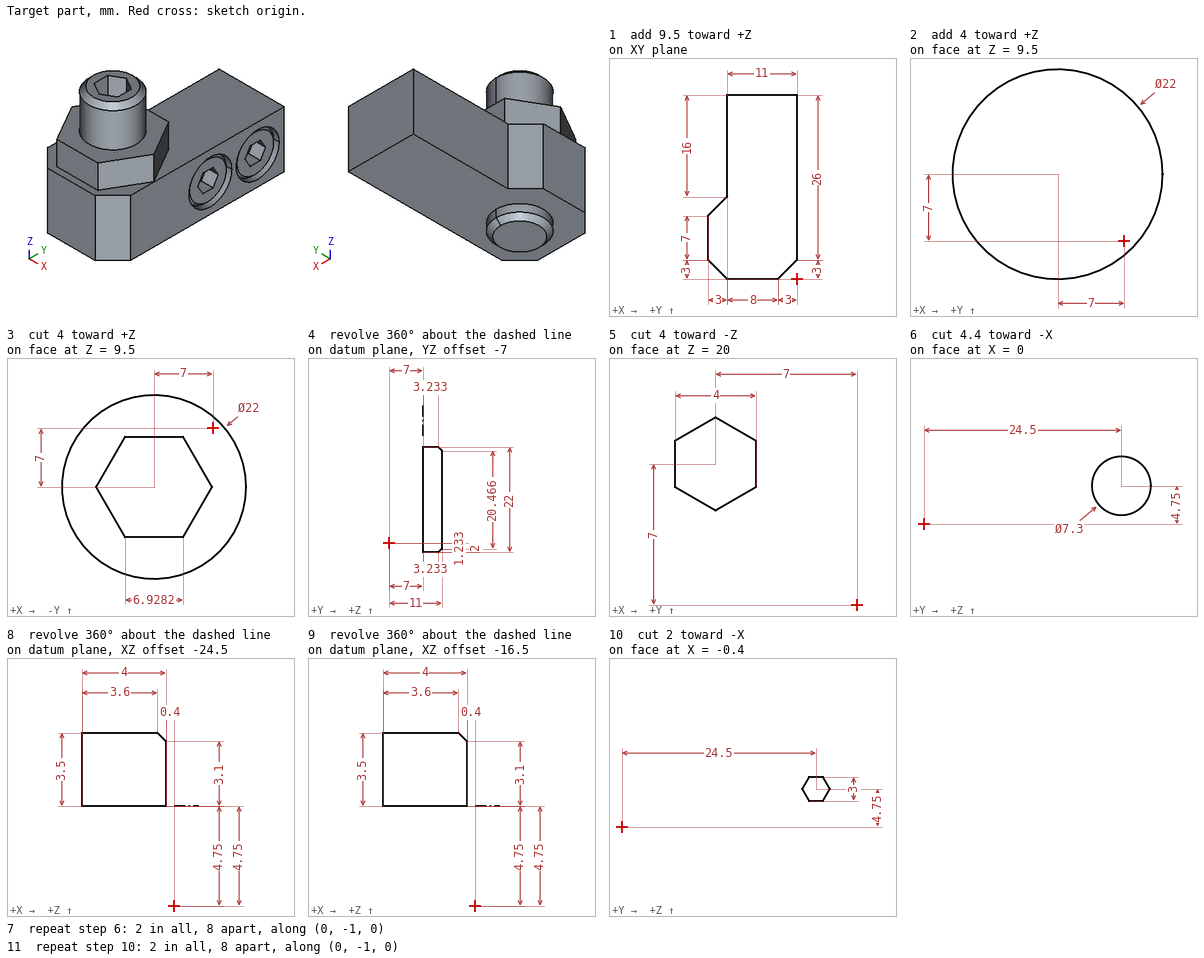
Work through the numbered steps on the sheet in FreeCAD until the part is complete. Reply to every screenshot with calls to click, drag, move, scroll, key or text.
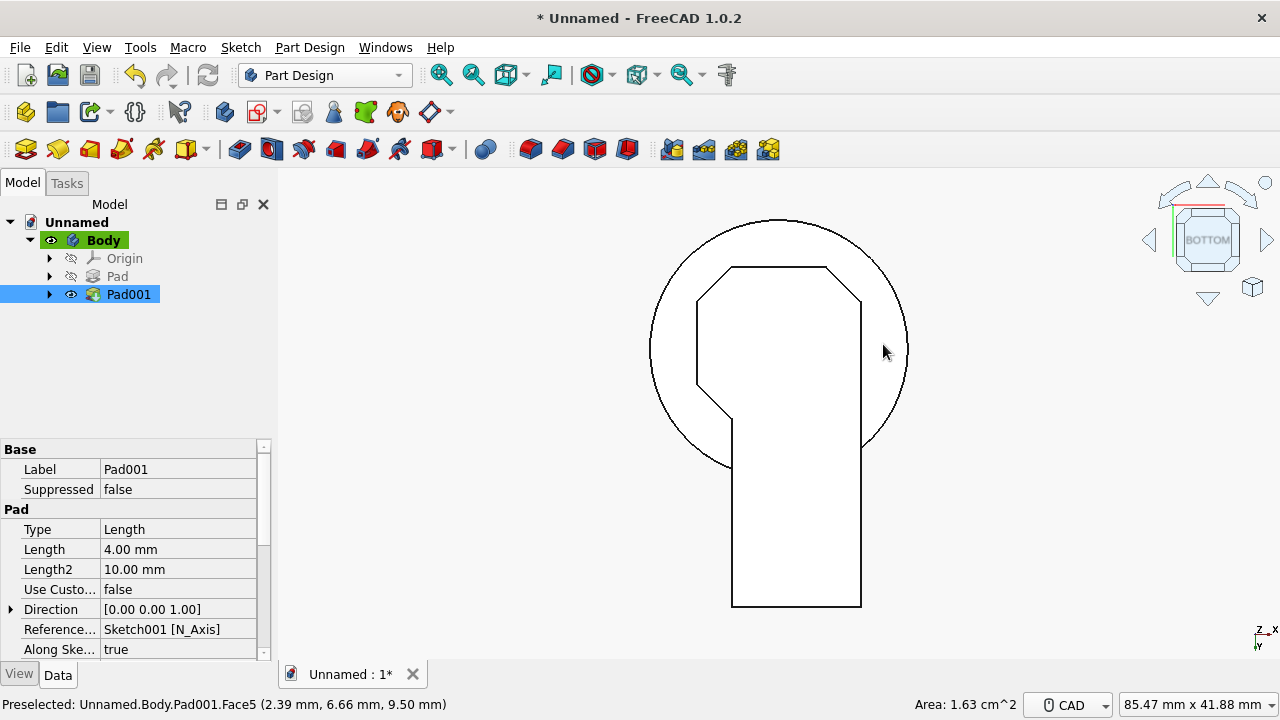
click(258, 112)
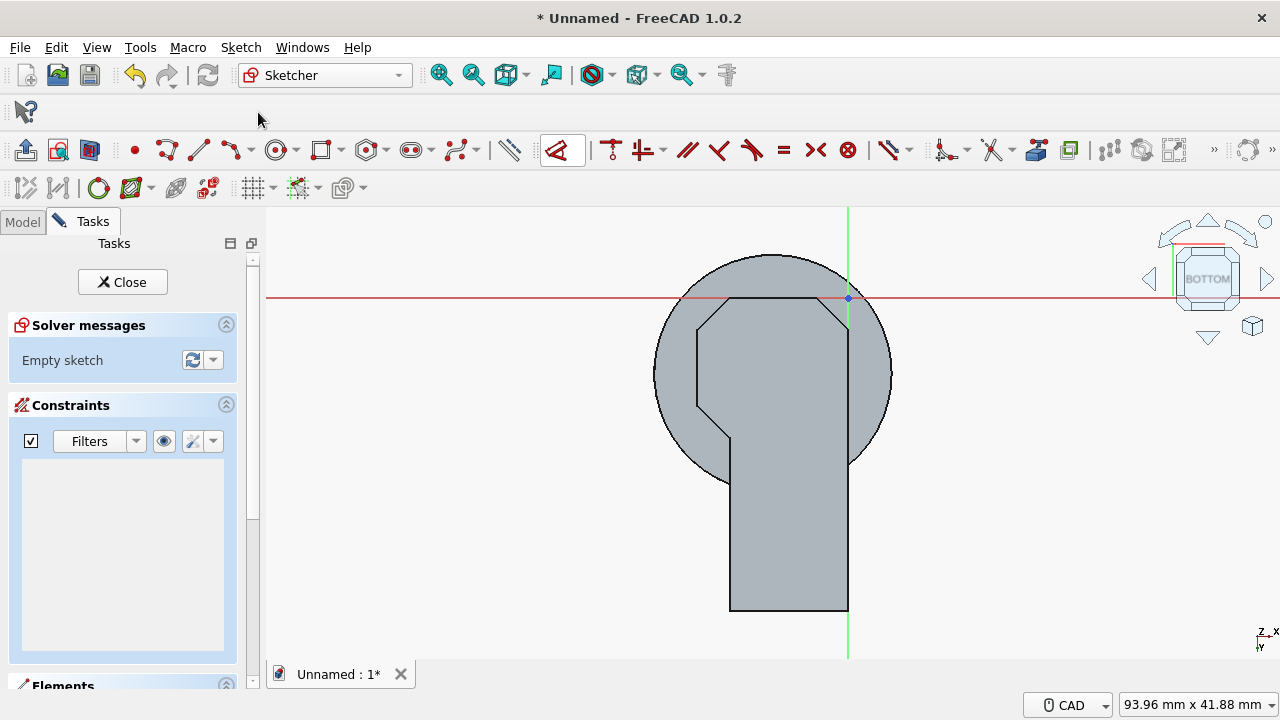
scroll(395, 631, down, 1)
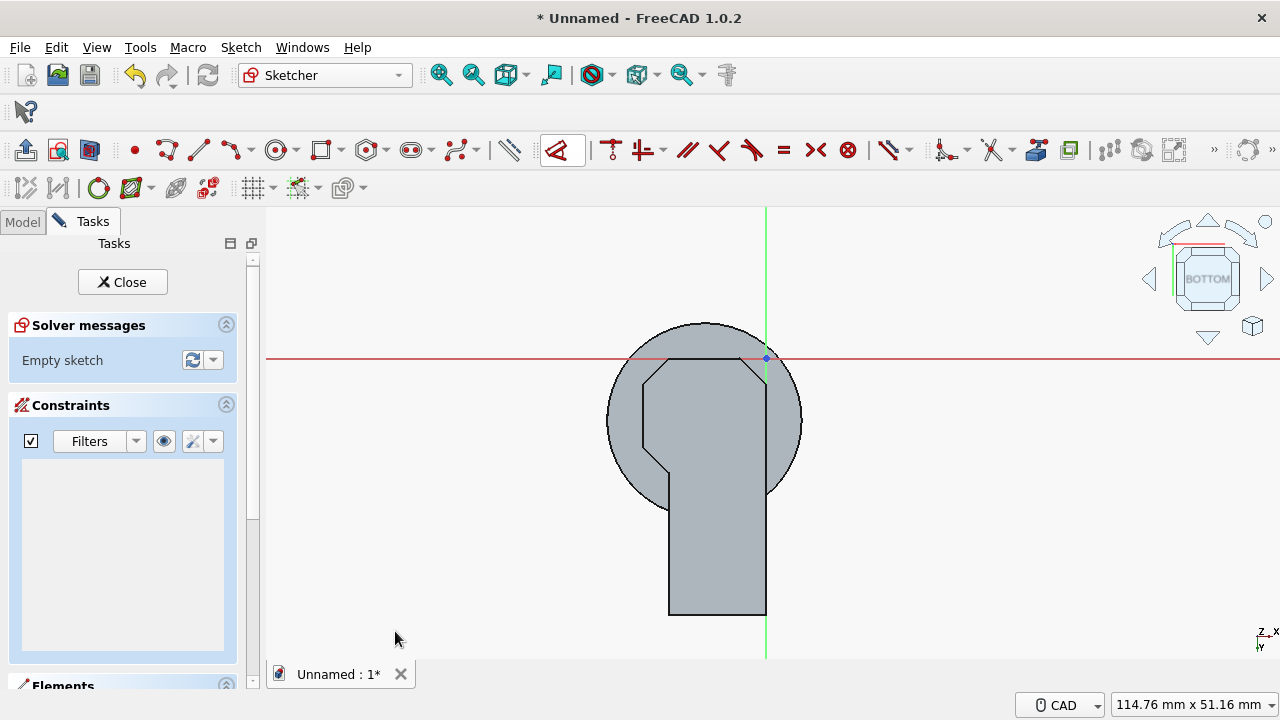
scroll(704, 395, up, 2)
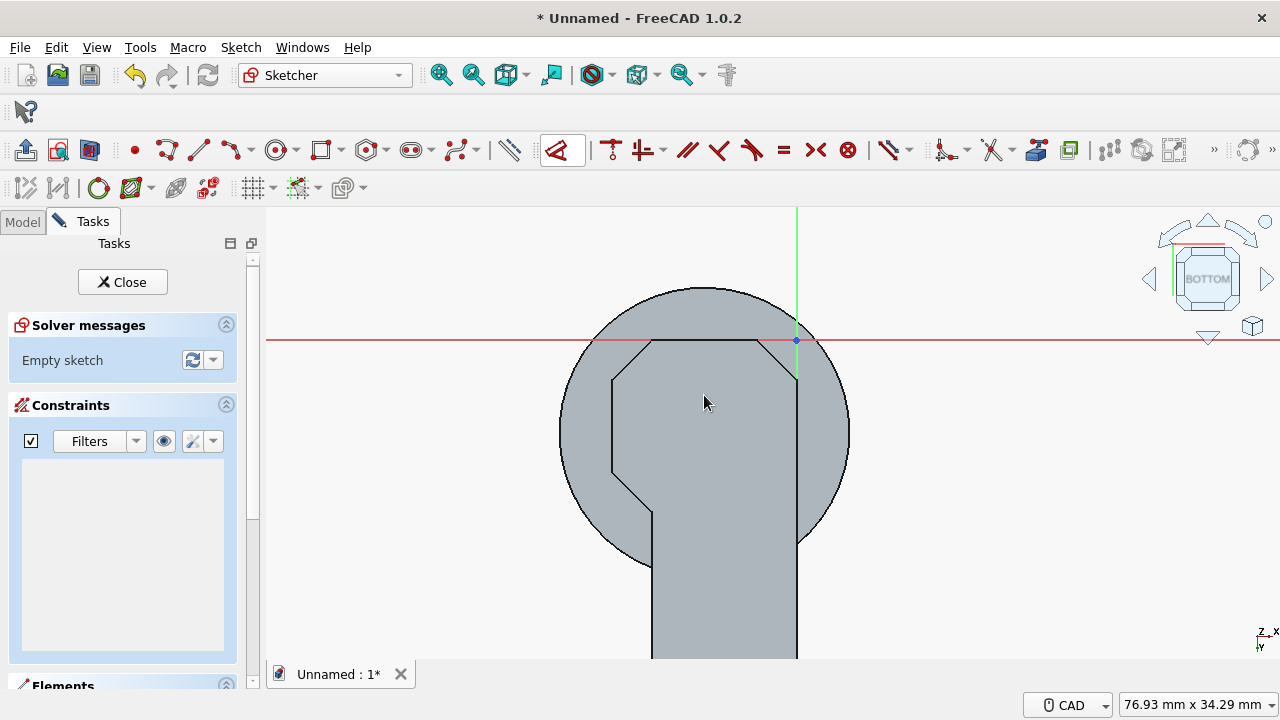
click(366, 150)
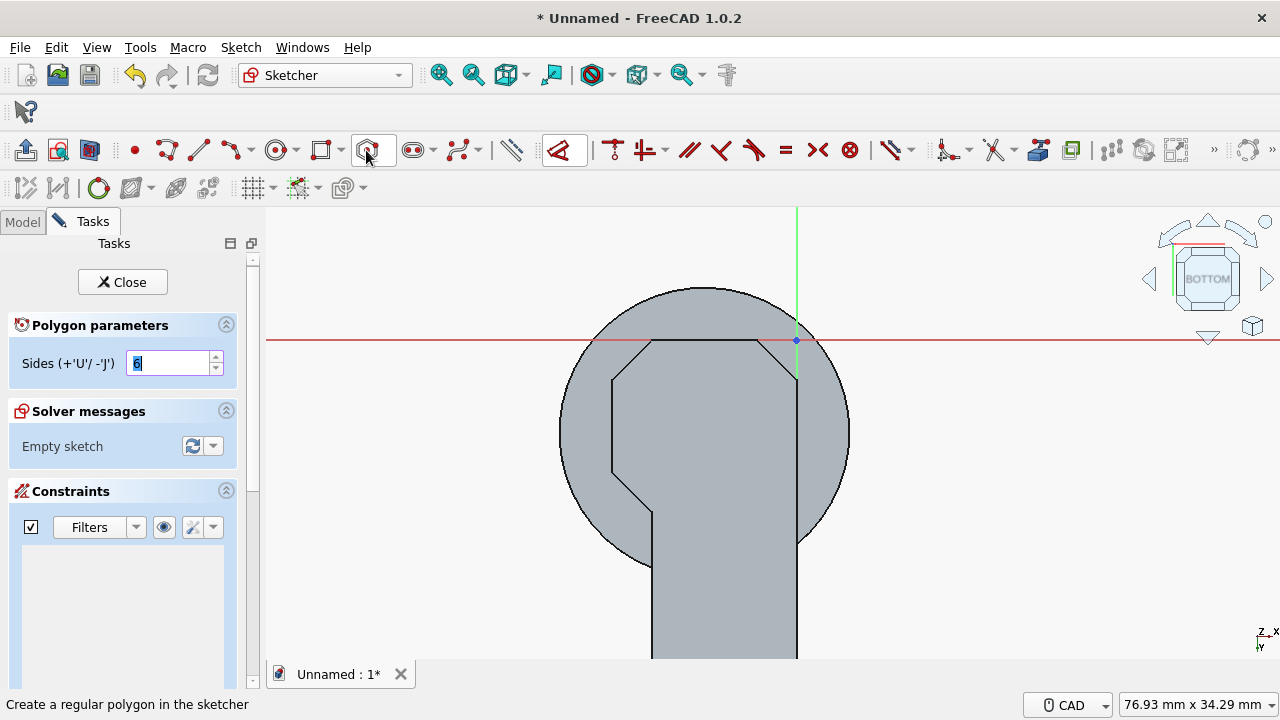
click(704, 433)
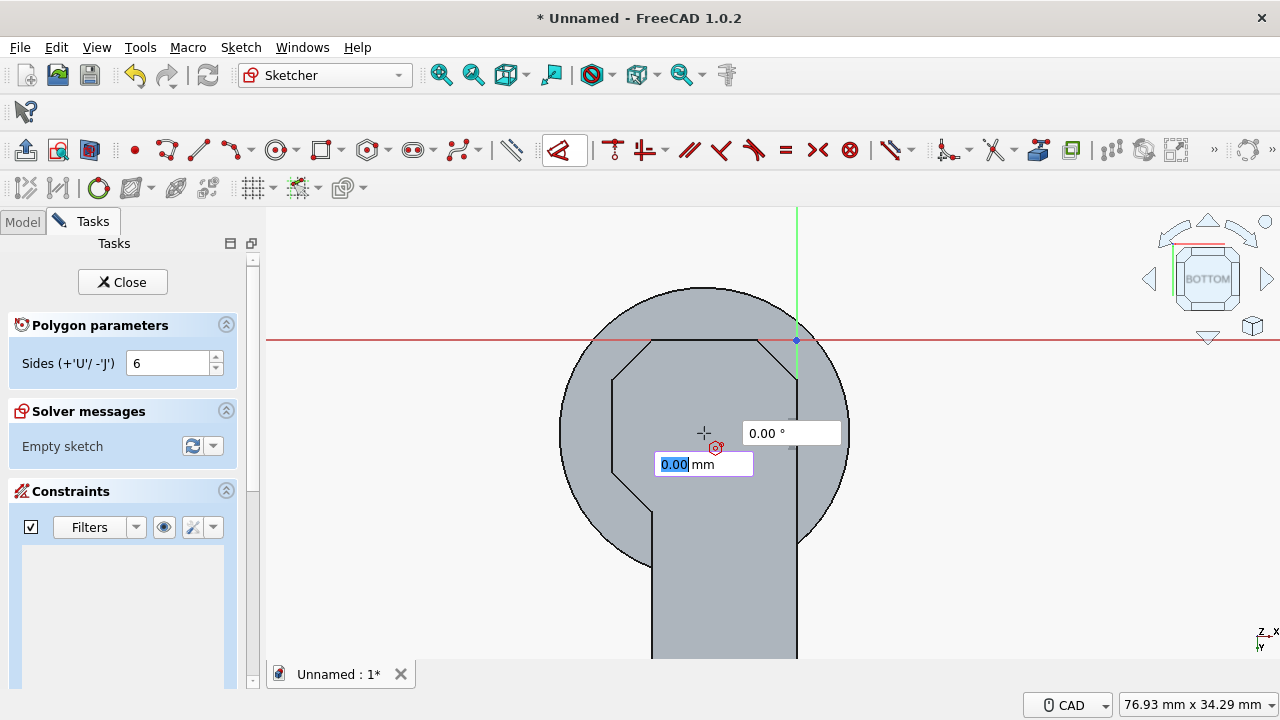
click(613, 433)
right_click(613, 433)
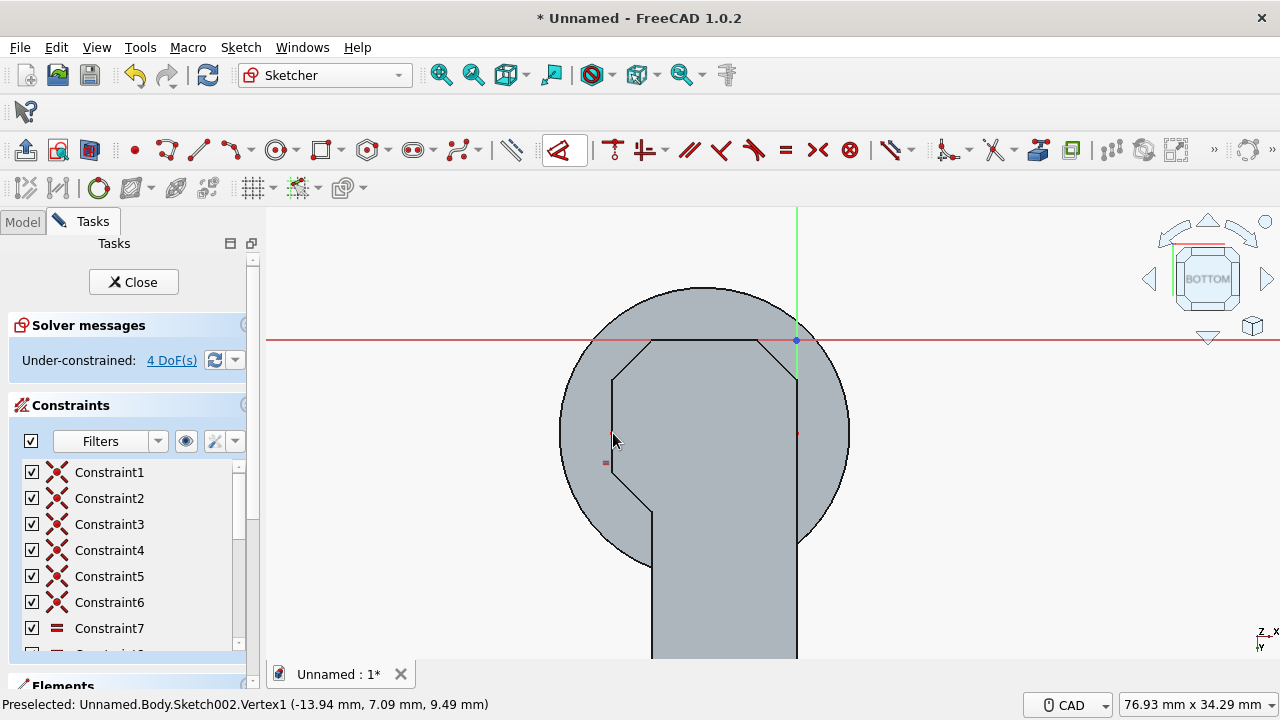
key(g)
key(c)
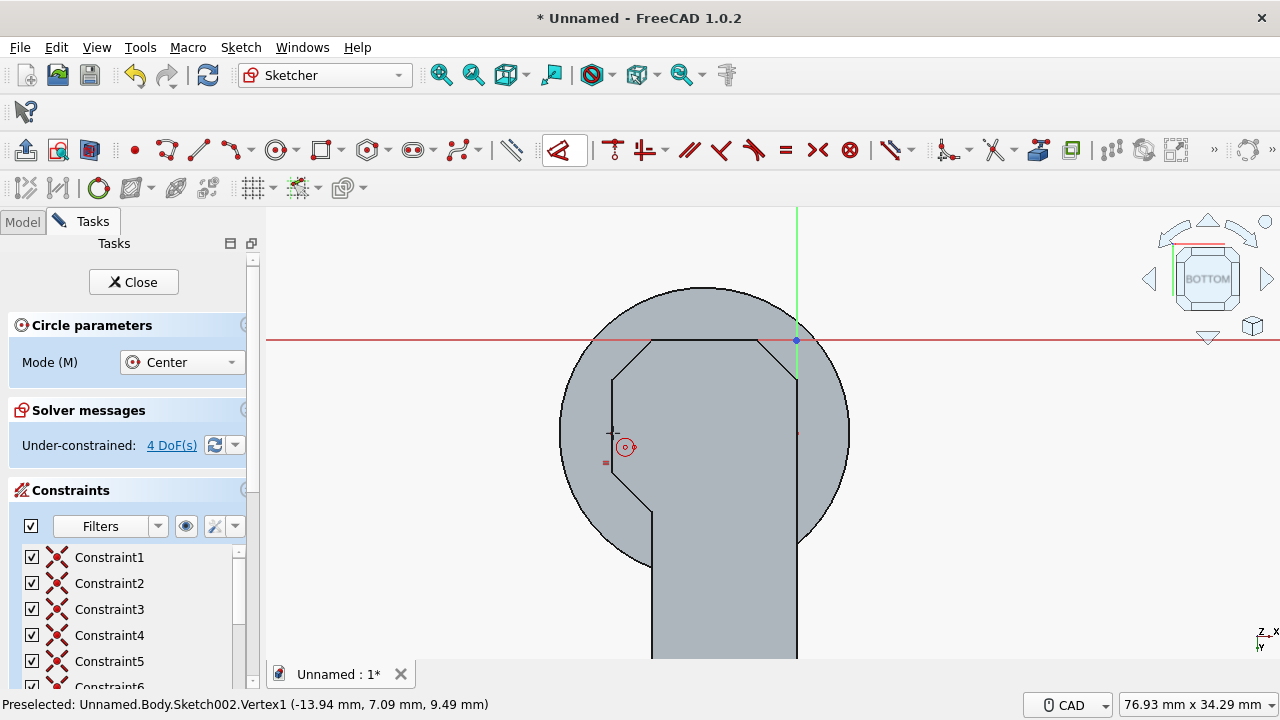
click(704, 434)
click(602, 535)
key(Escape)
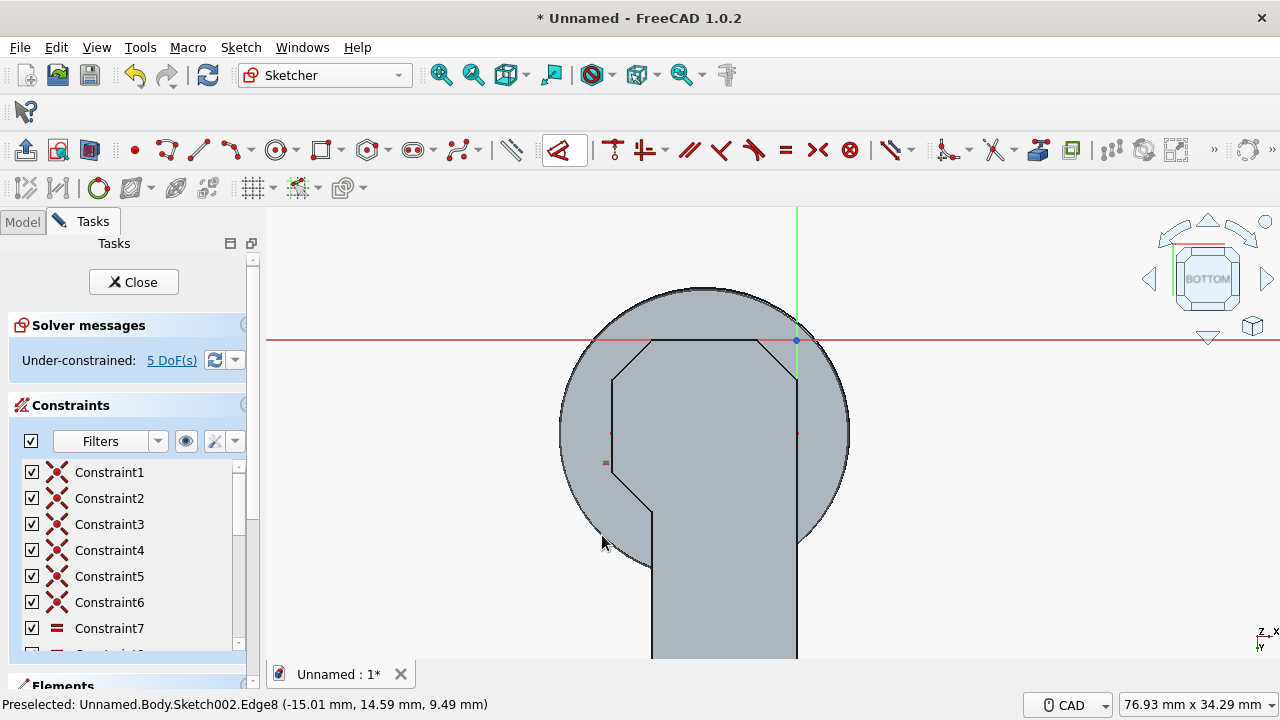
scroll(686, 513, up, 2)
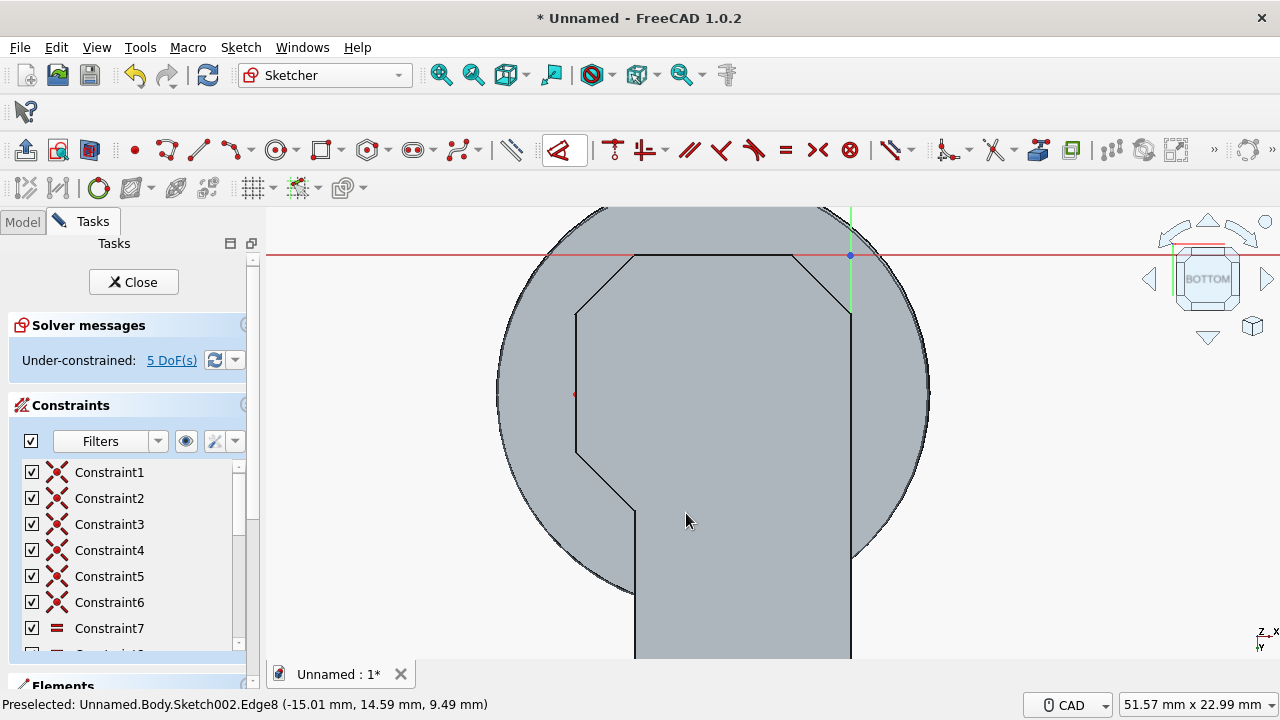
click(685, 512)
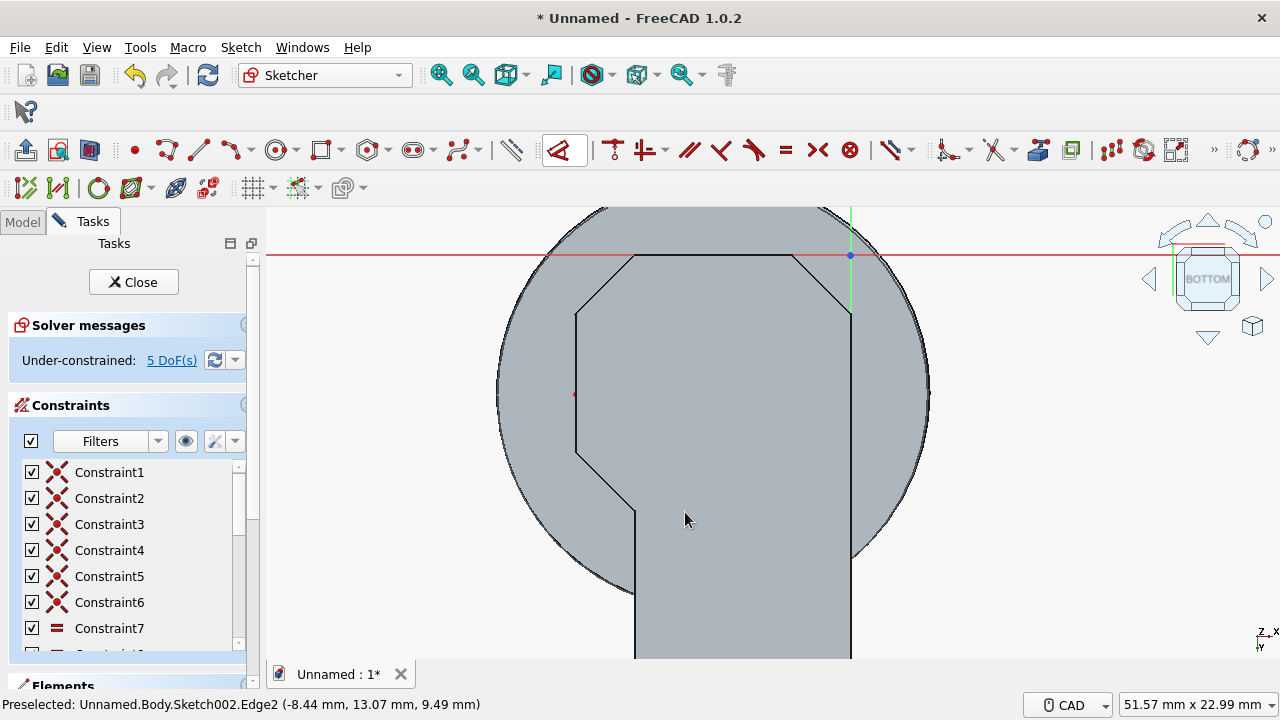
key(h)